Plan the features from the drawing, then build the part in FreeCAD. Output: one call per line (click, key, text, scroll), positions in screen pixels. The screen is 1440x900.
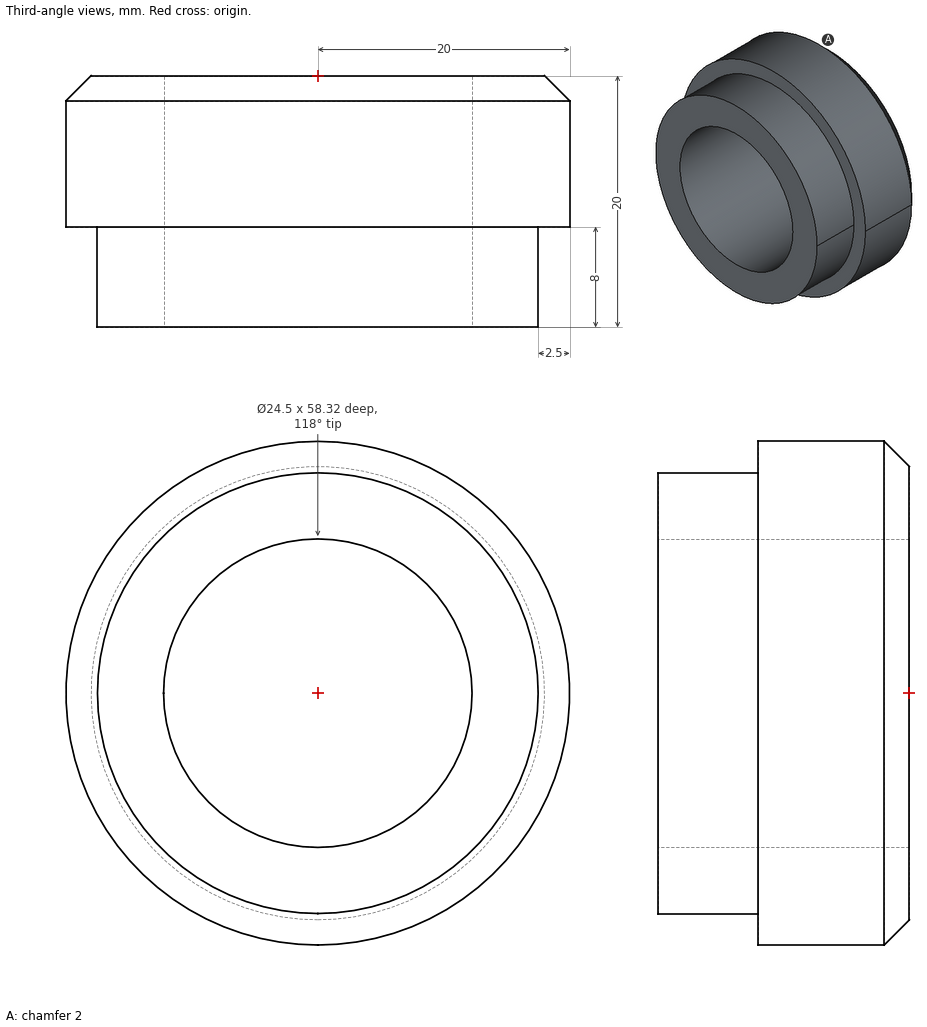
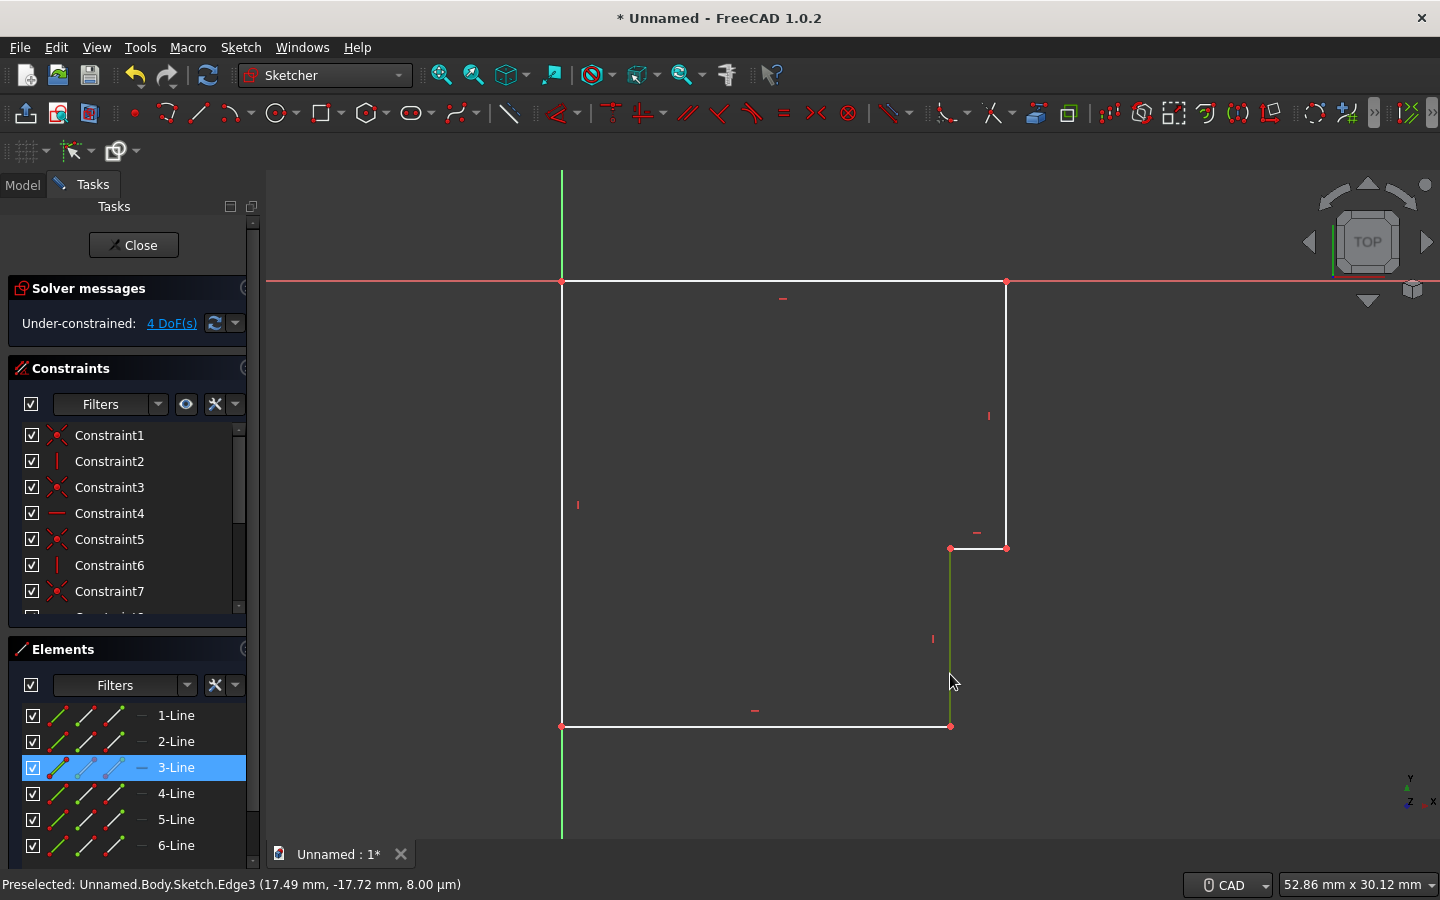
click(580, 114)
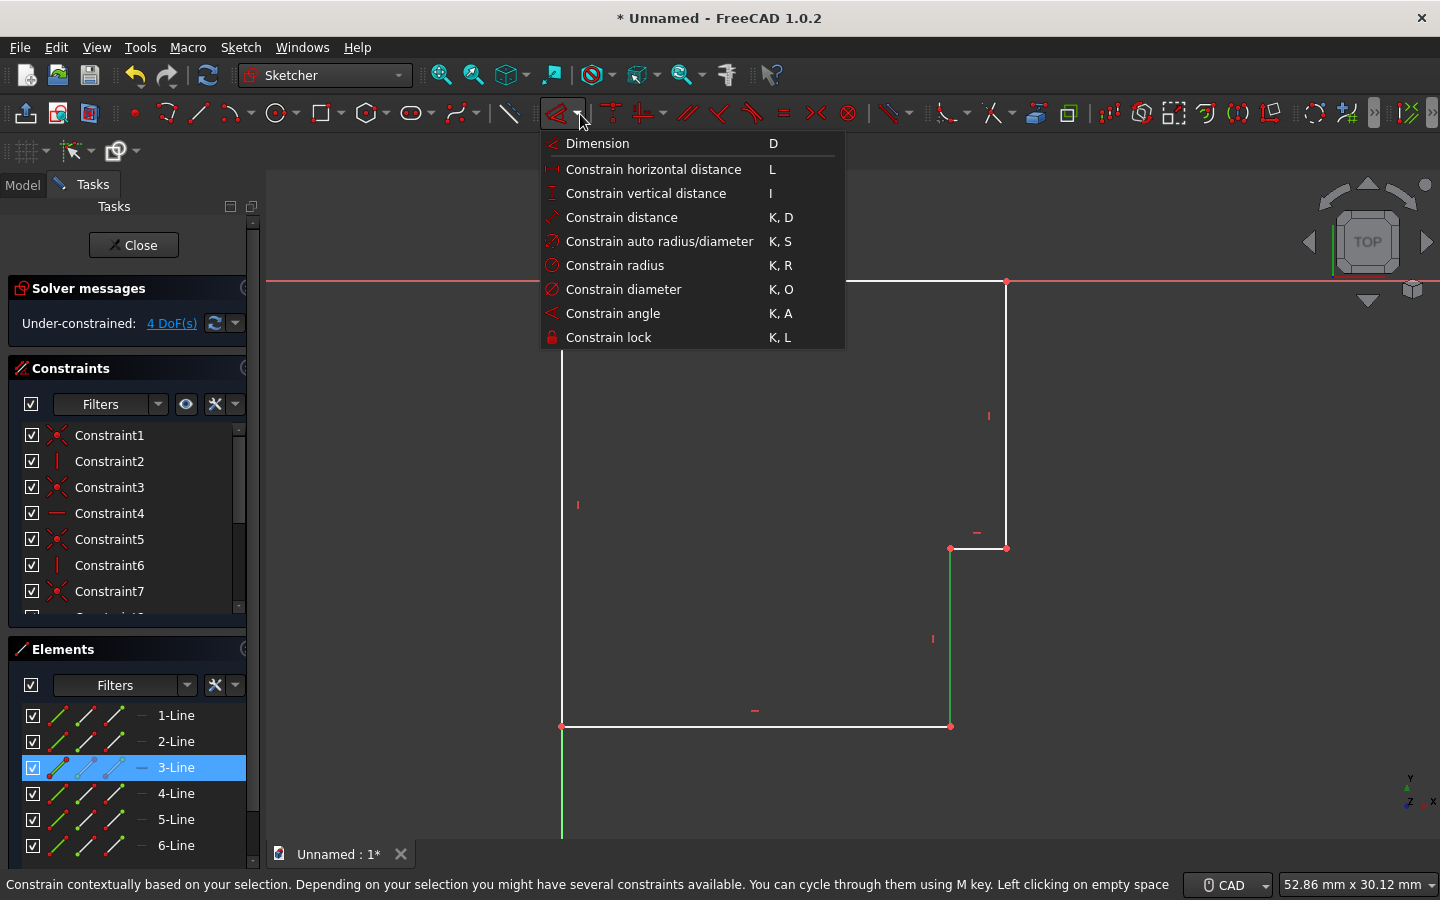
click(693, 193)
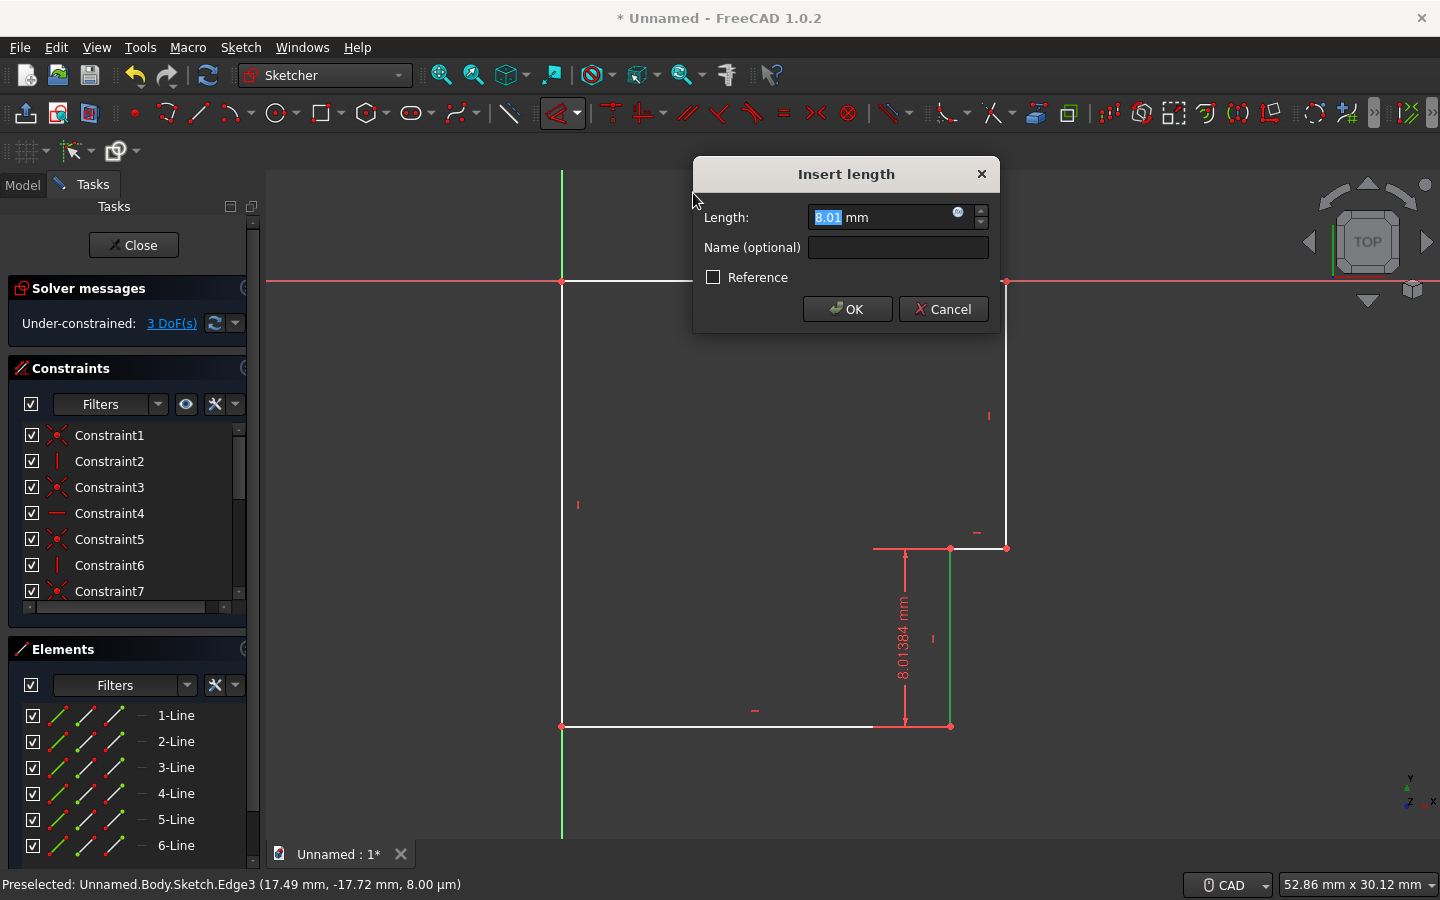
text(8)
key(Return)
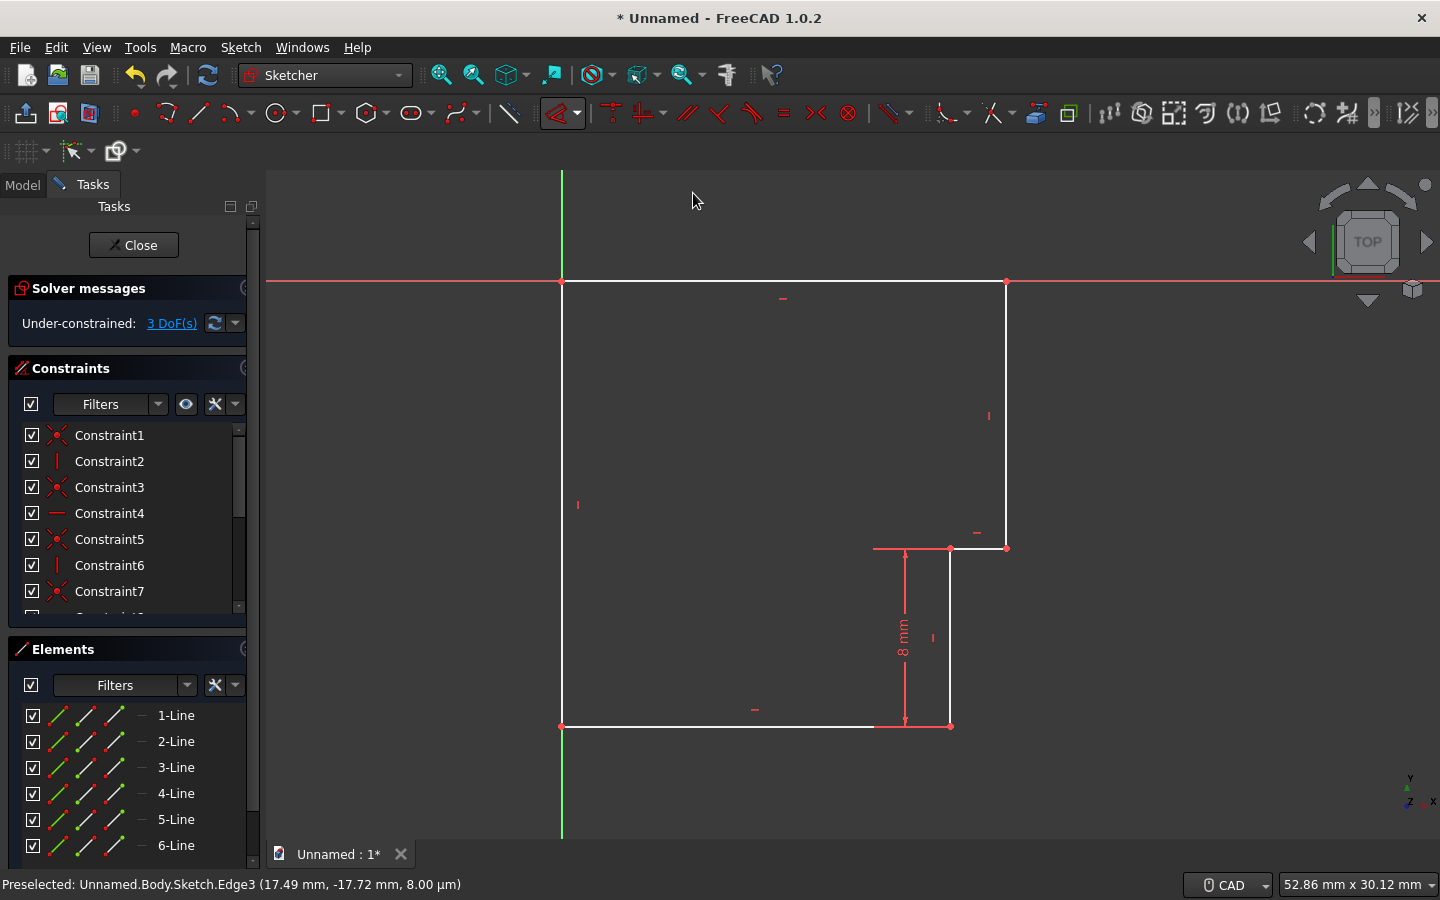
click(562, 415)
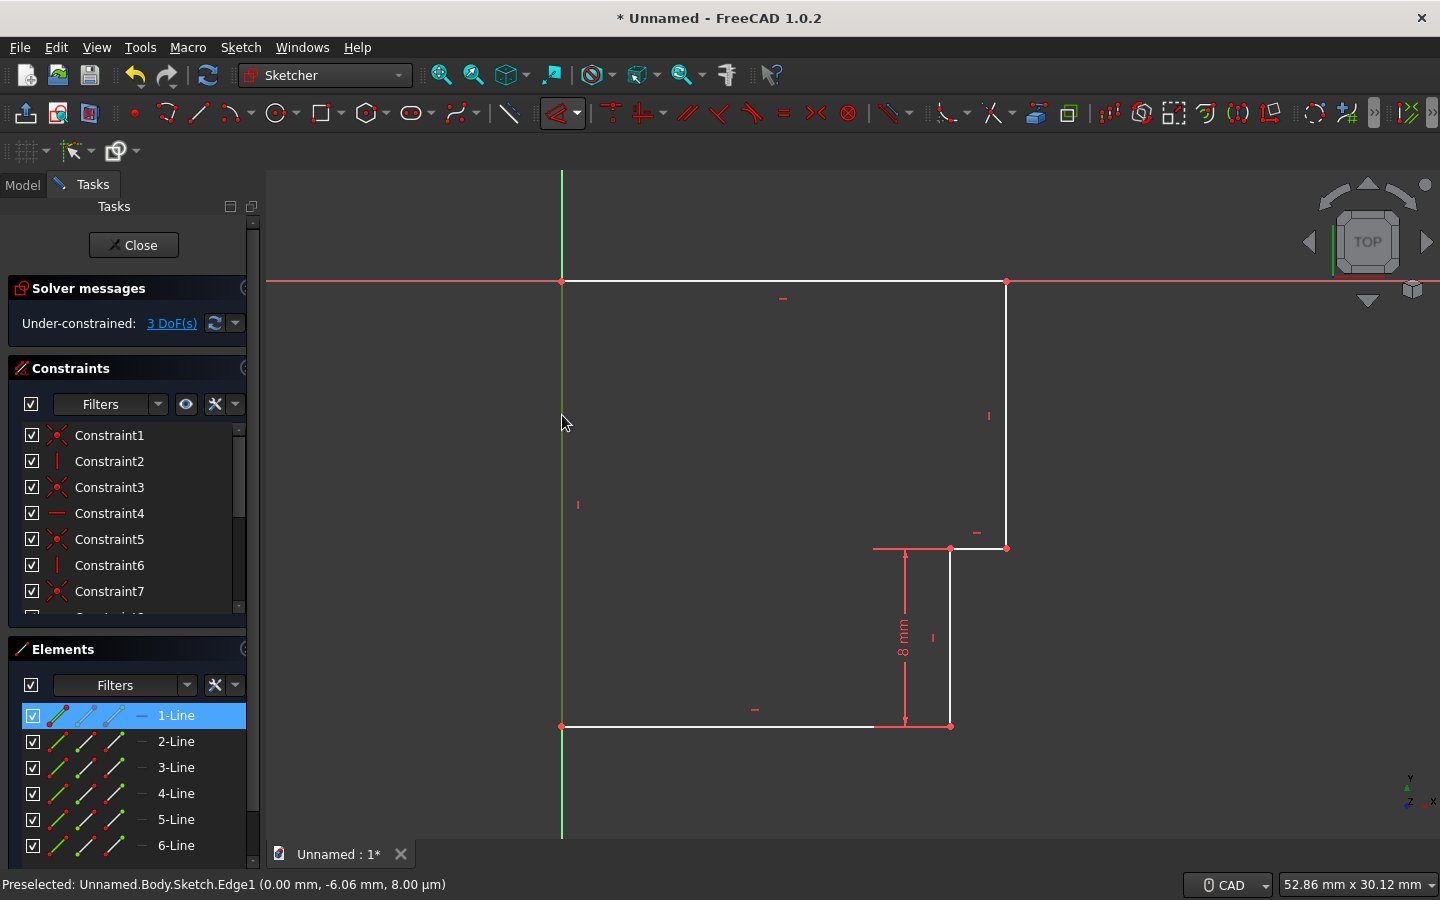
key(i)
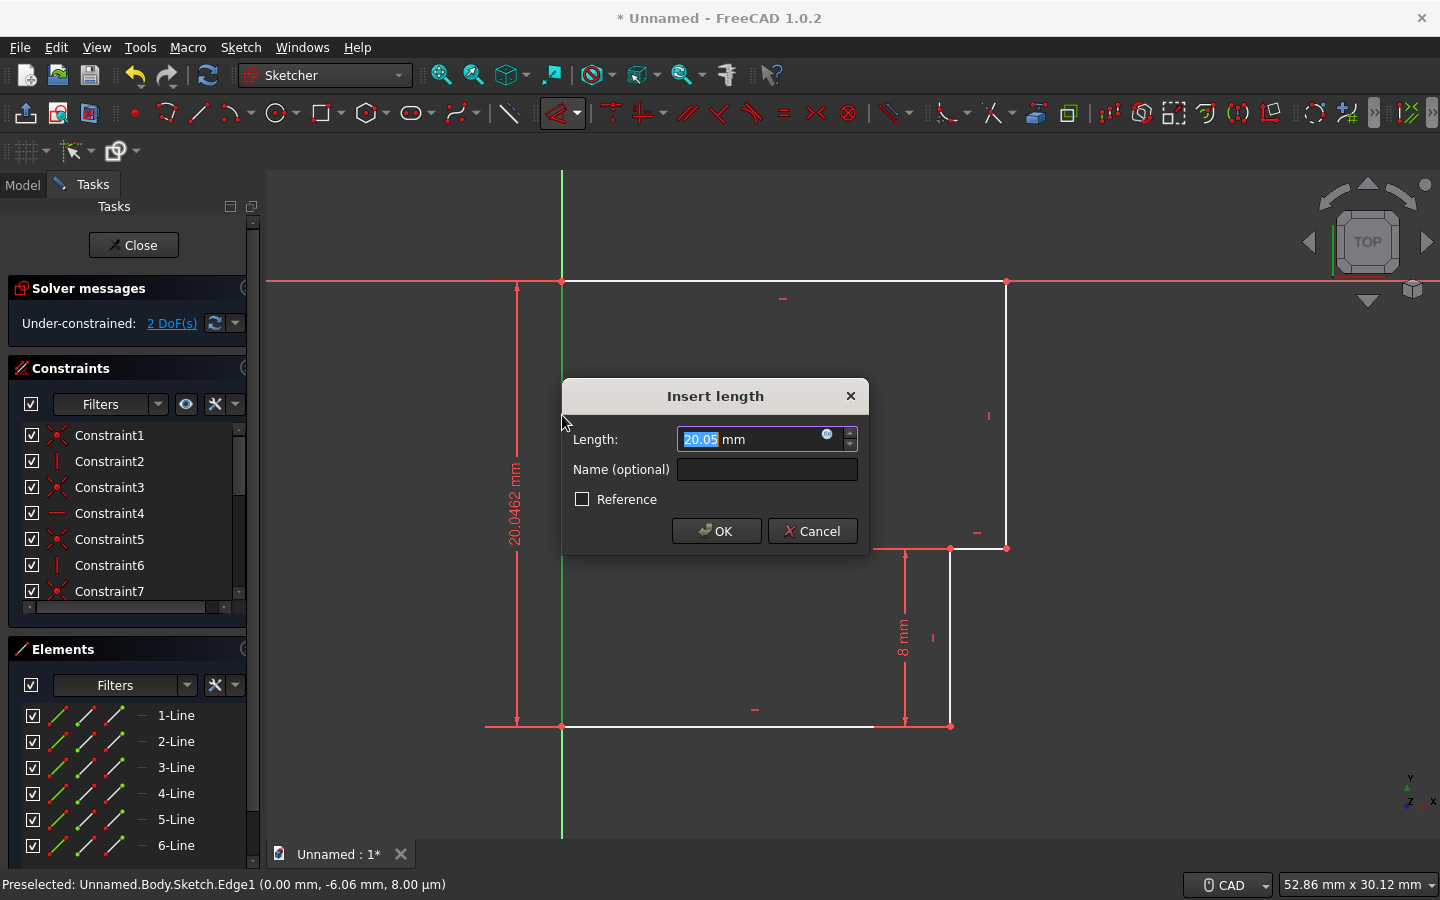
text(20)
key(Return)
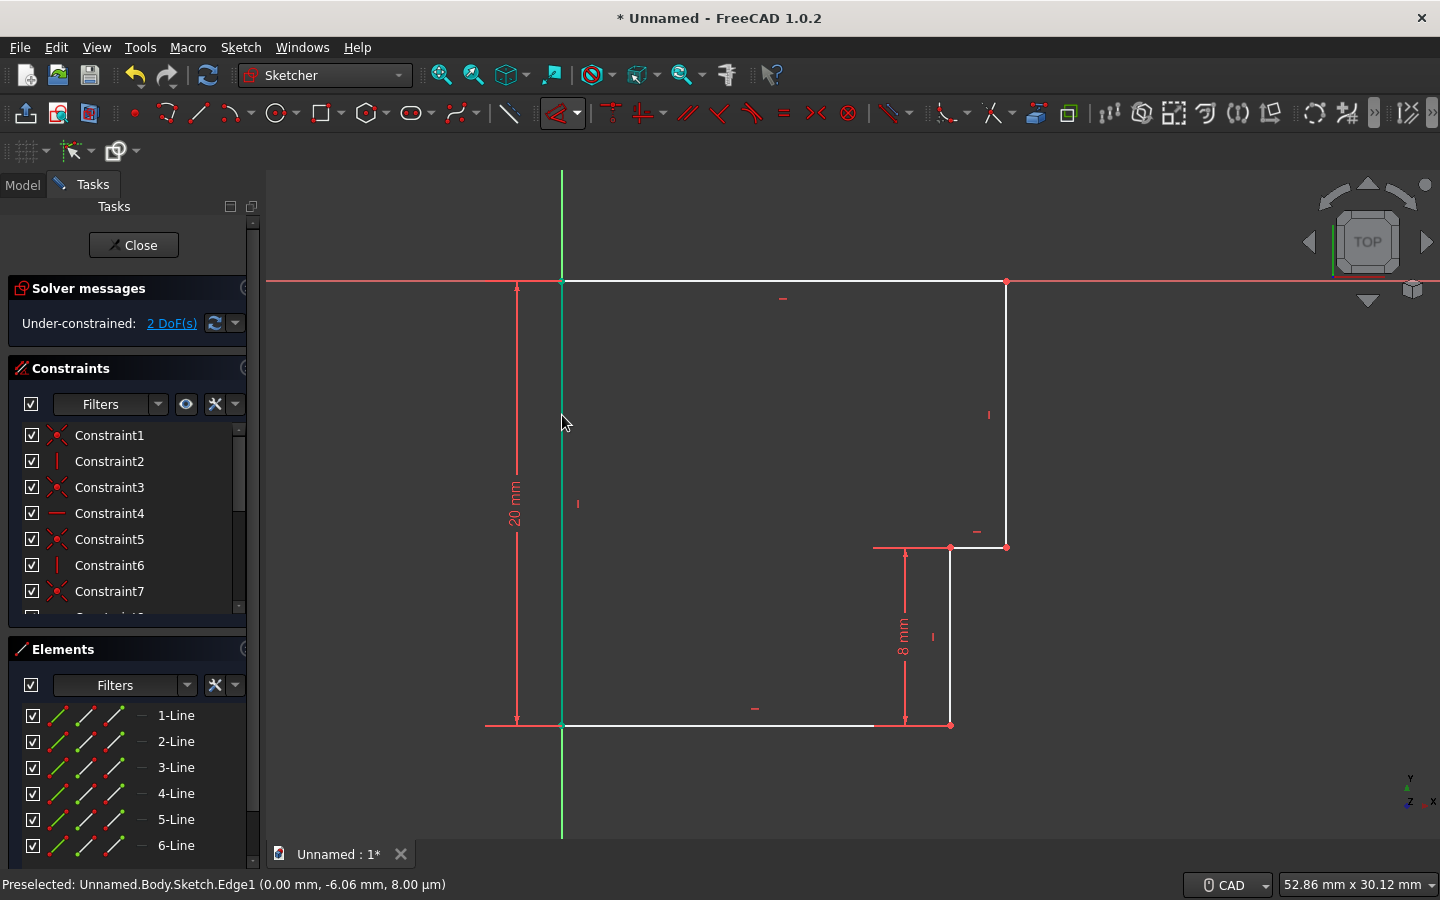
click(873, 281)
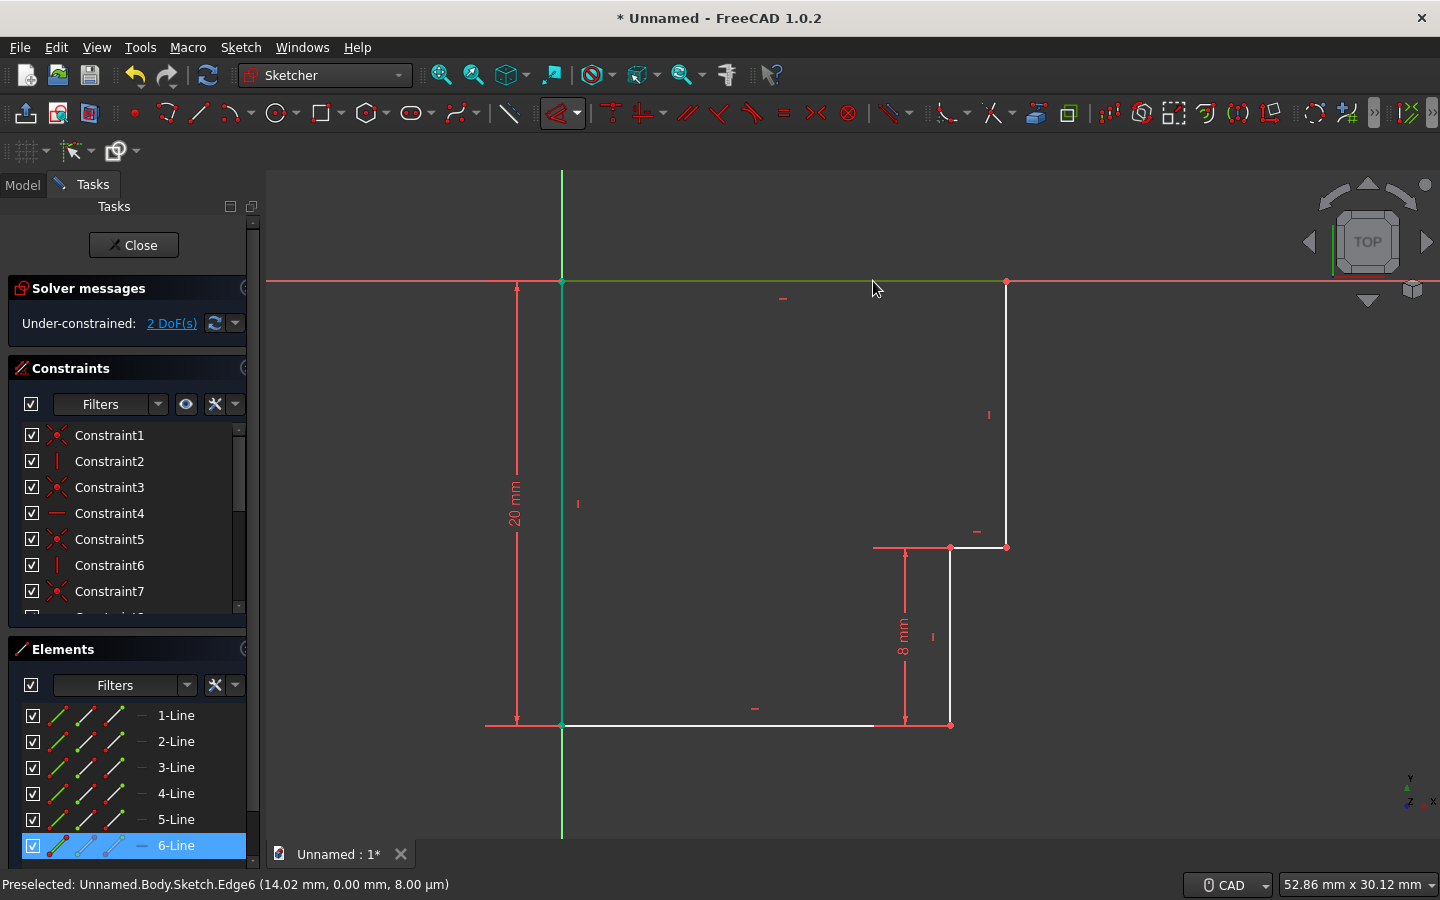
click(580, 114)